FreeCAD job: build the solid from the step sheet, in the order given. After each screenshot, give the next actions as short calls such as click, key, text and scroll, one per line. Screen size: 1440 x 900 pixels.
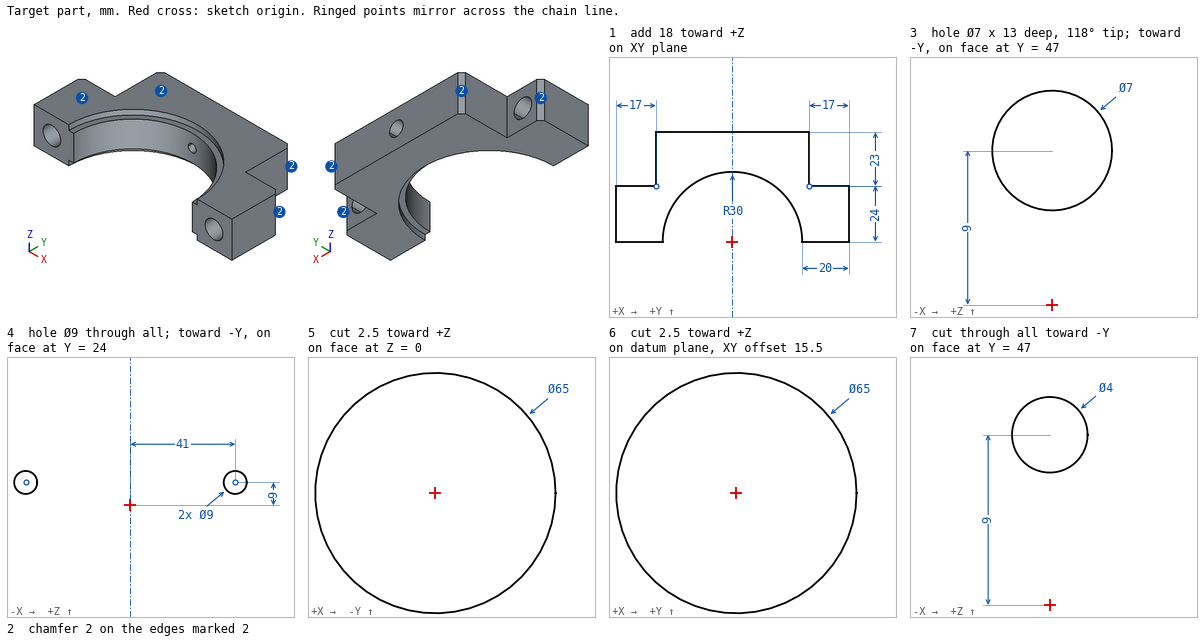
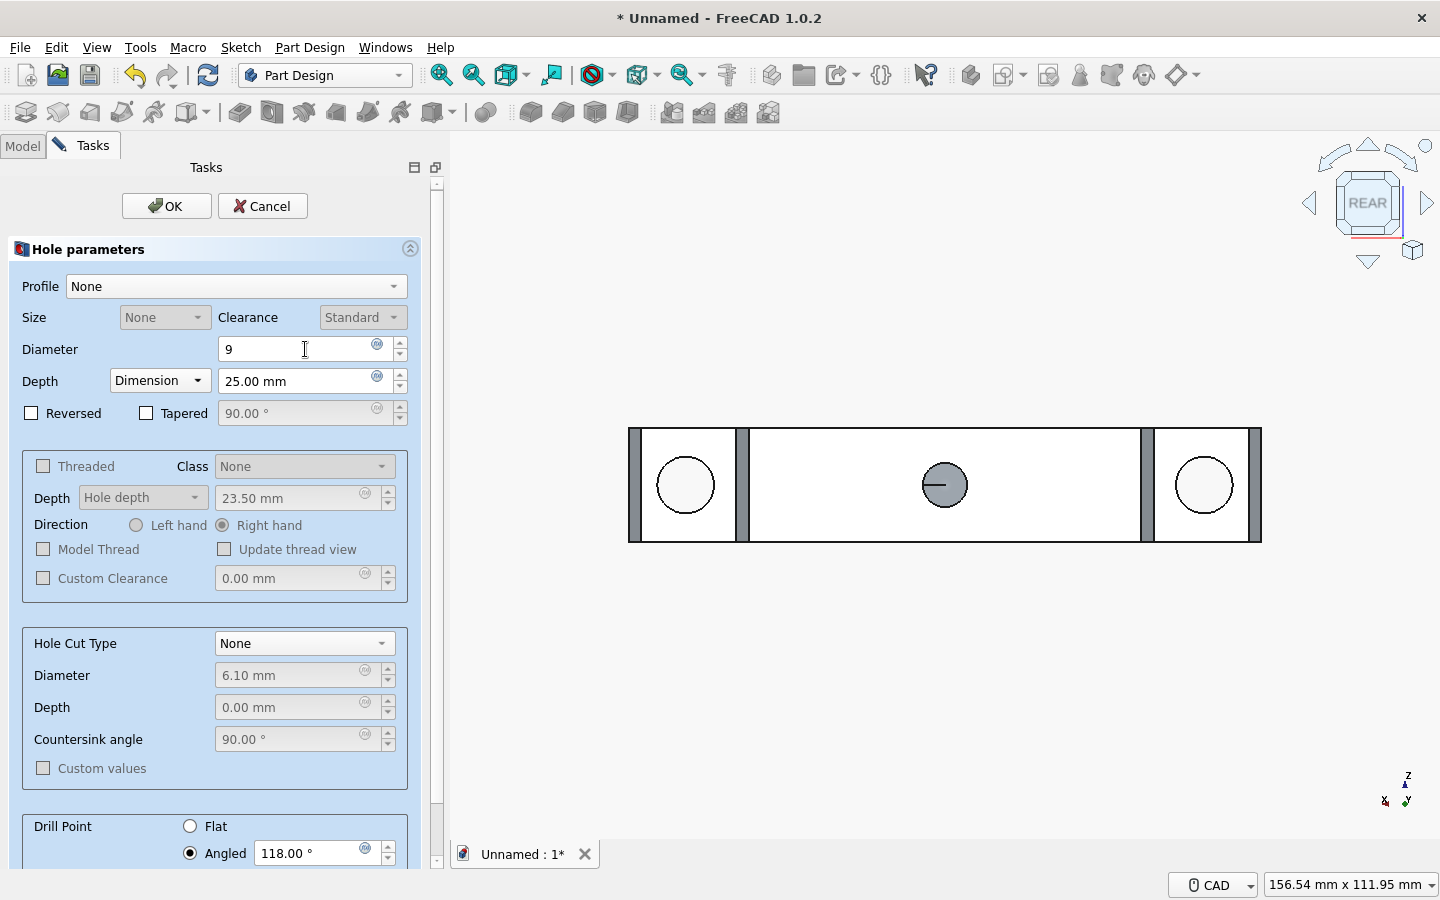
click(161, 380)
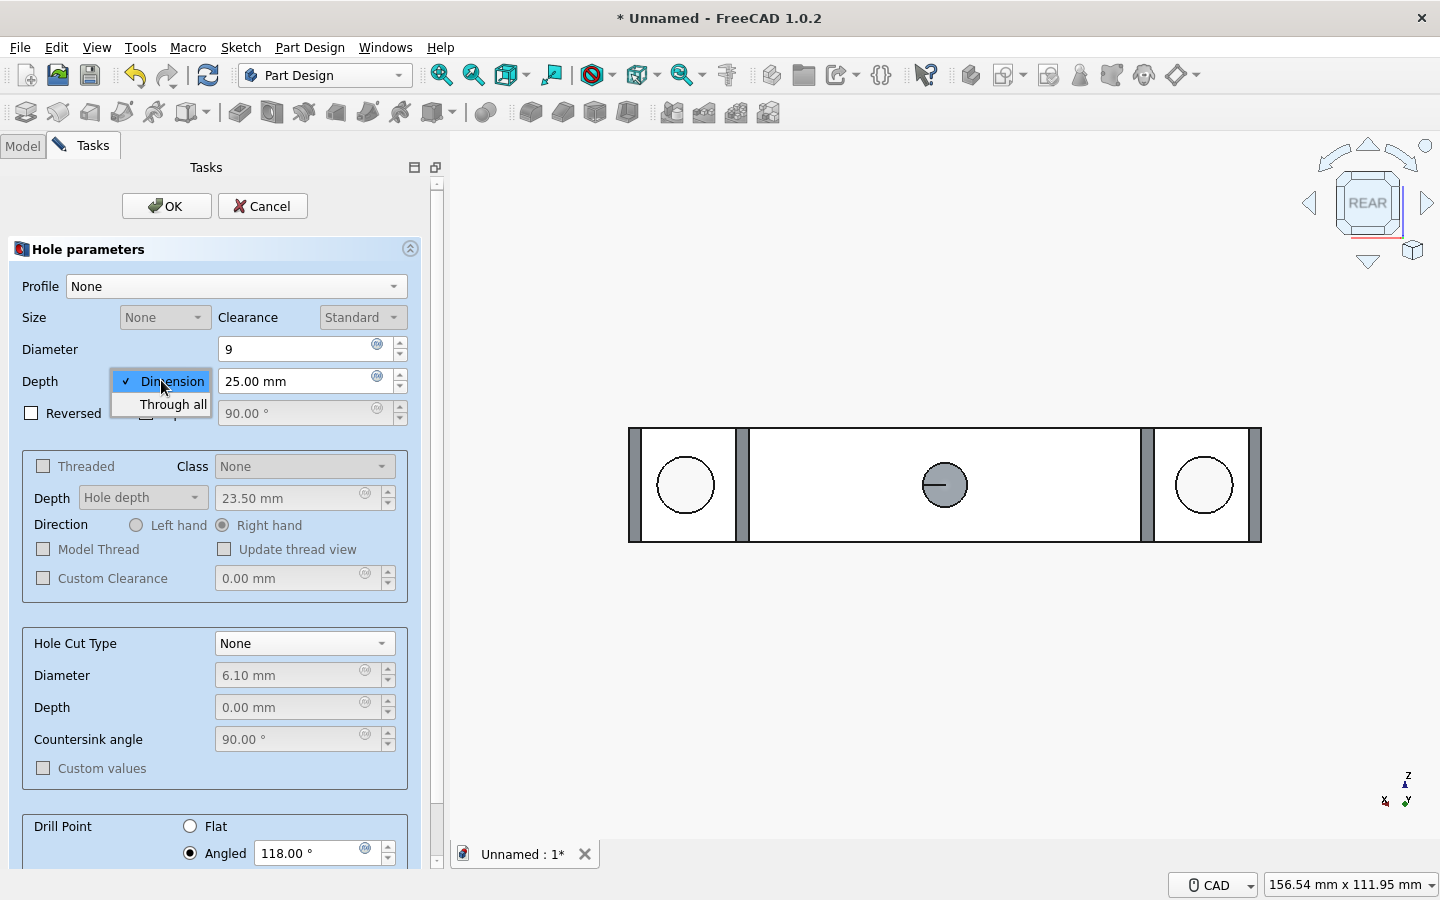
click(160, 404)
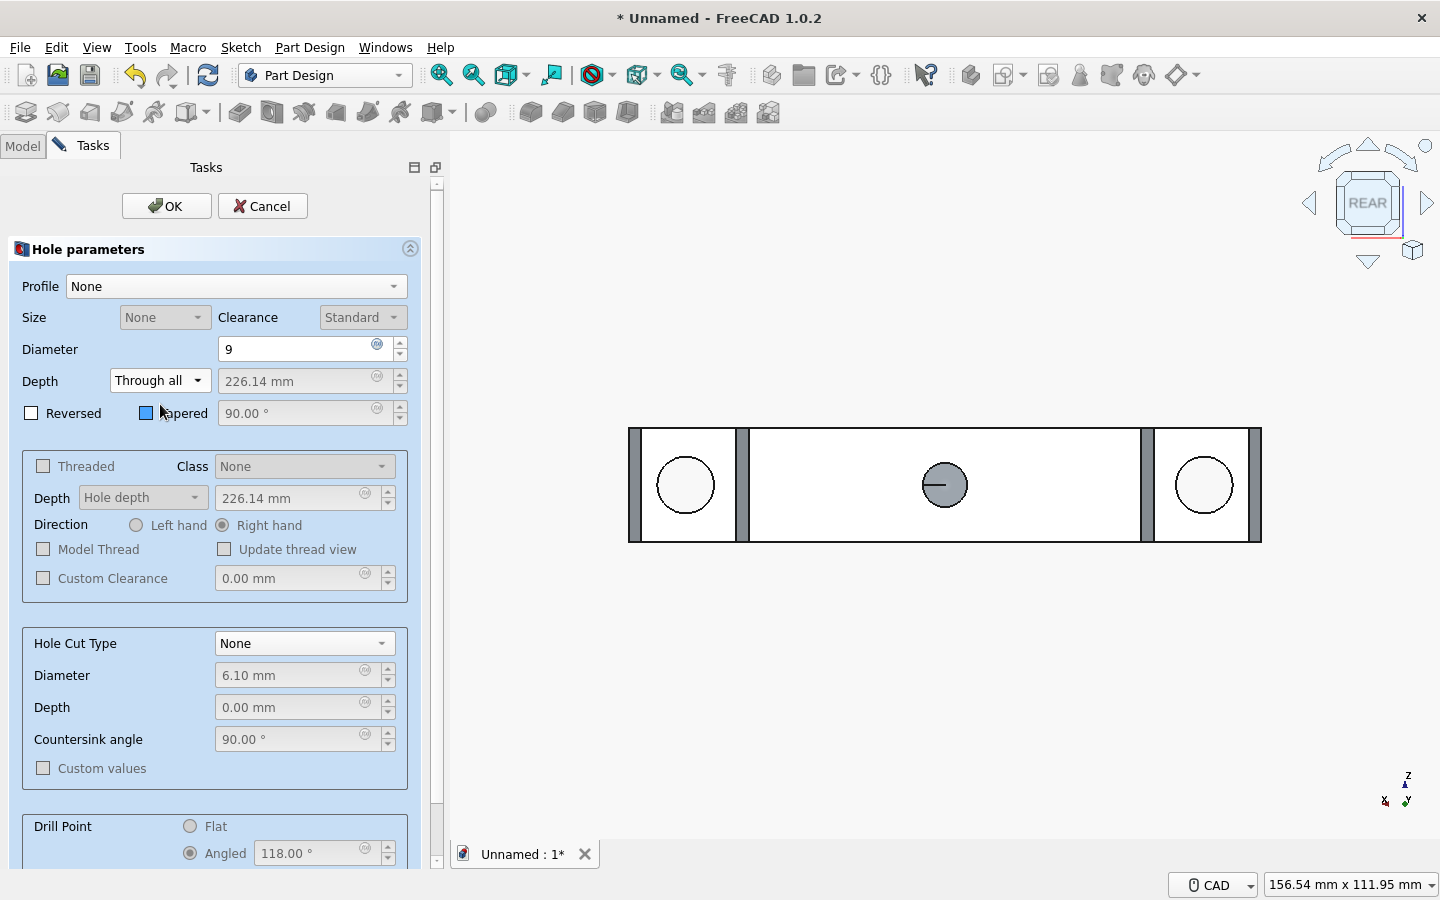
click(167, 206)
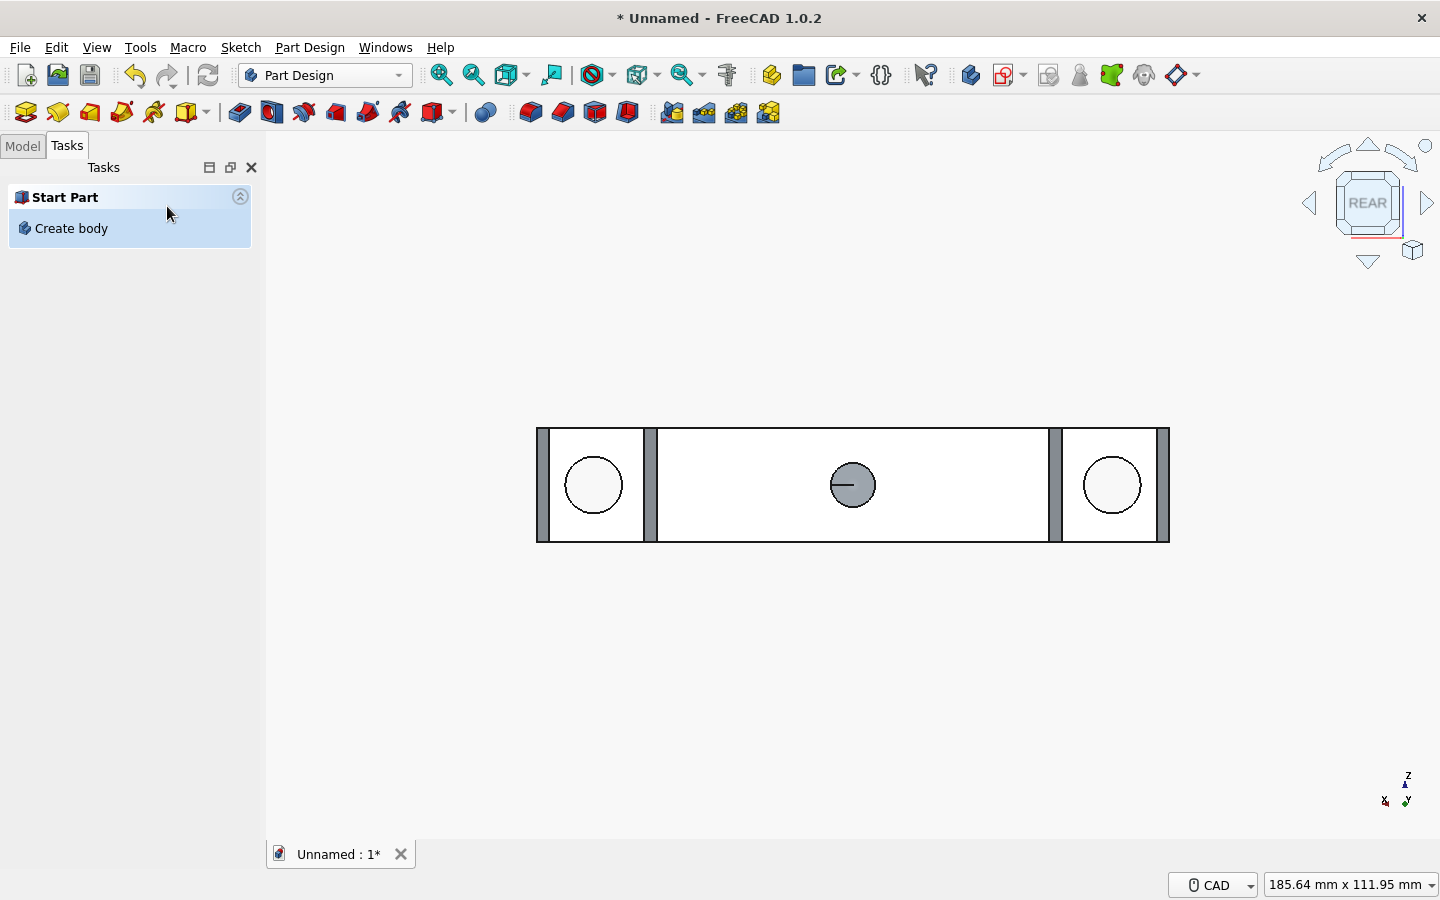
key(5)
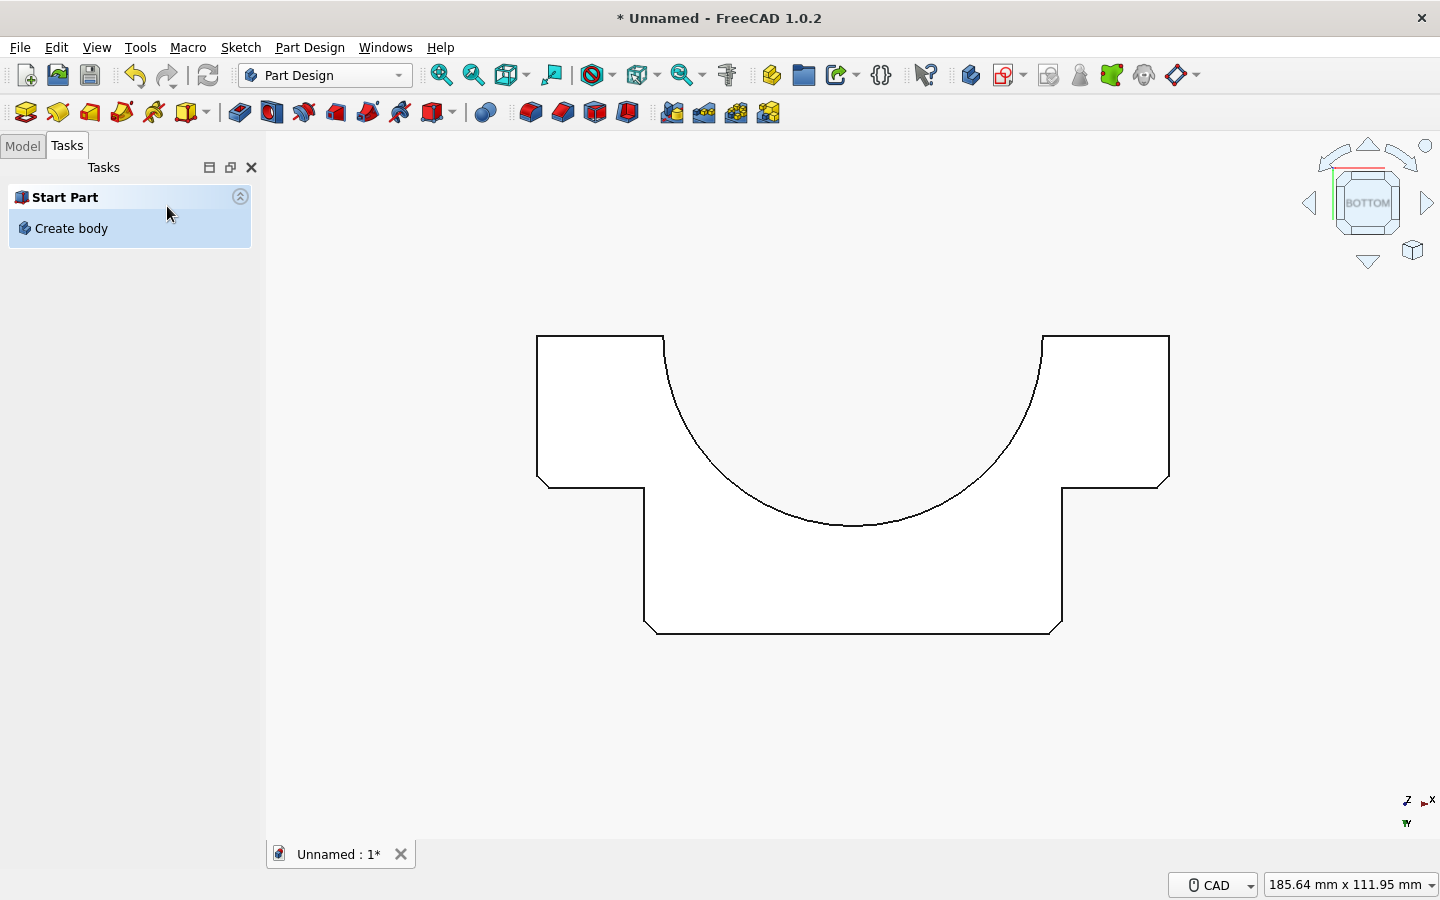
click(943, 569)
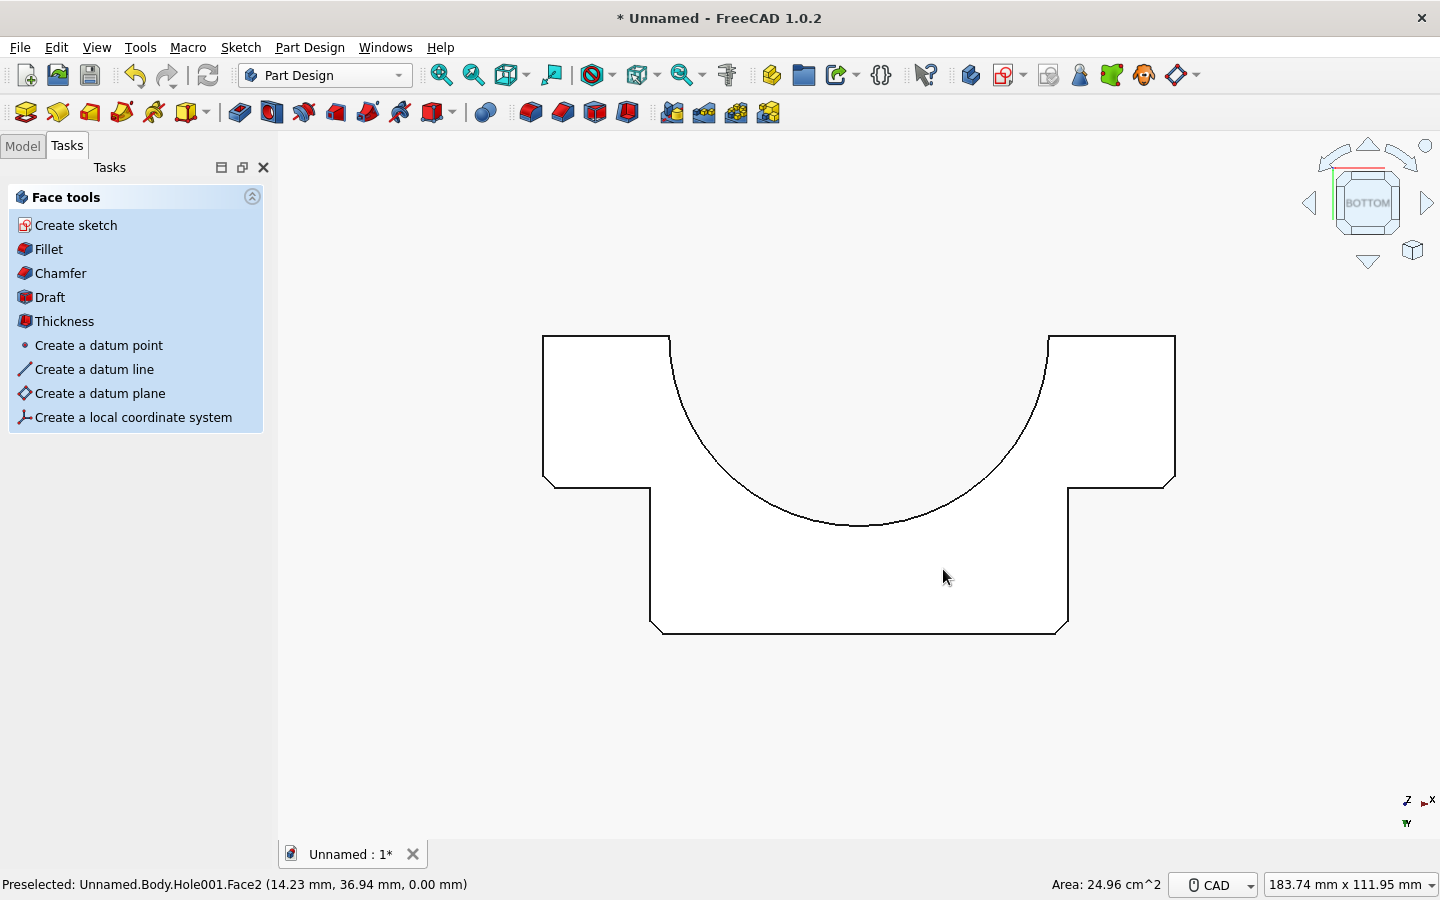
click(1004, 76)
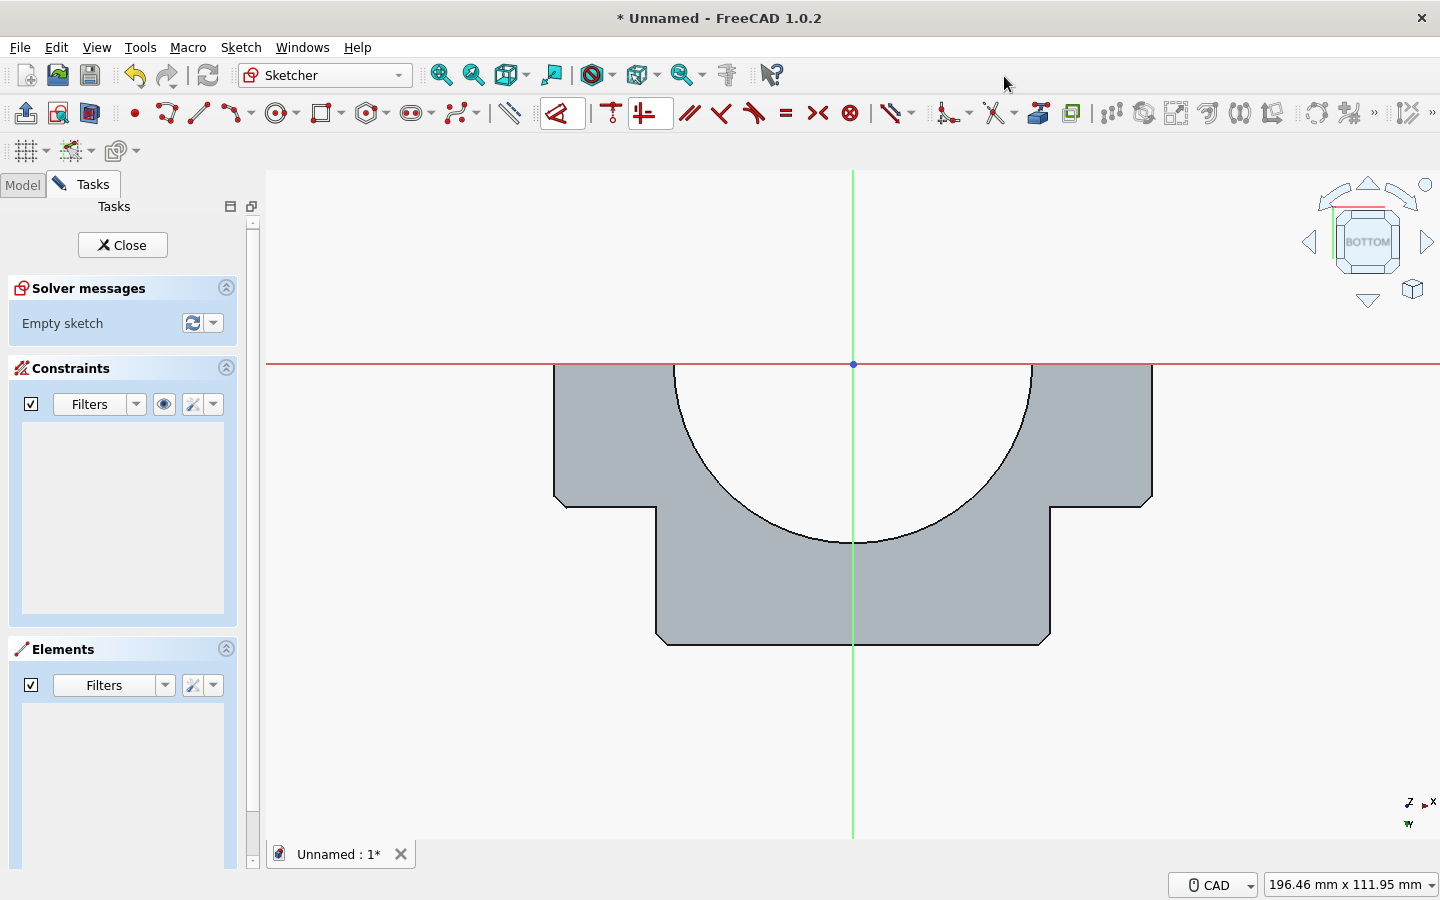
scroll(475, 811, down, 1)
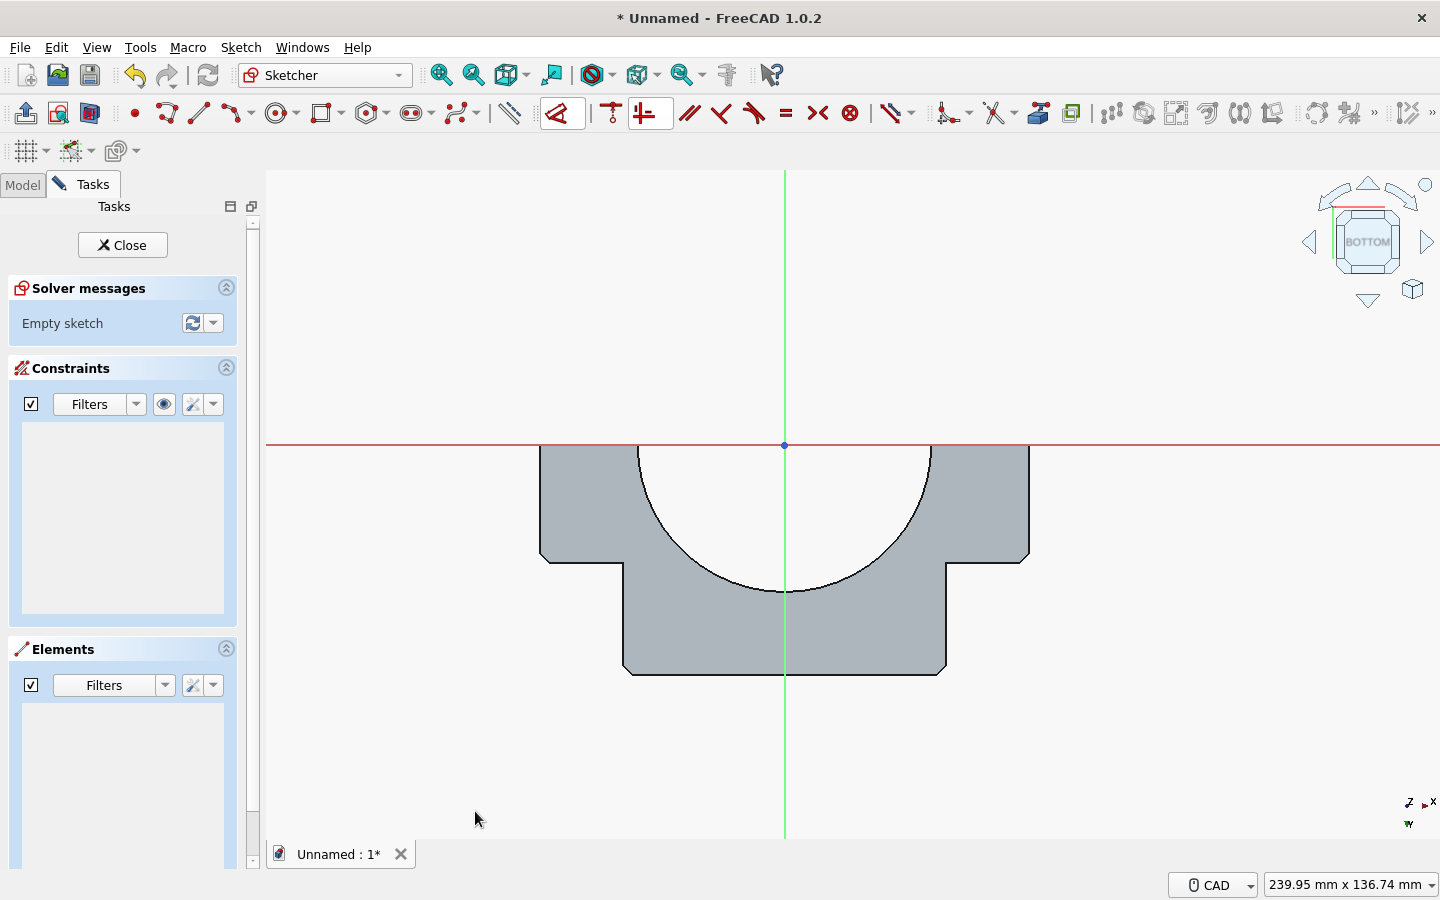
scroll(785, 325, up, 2)